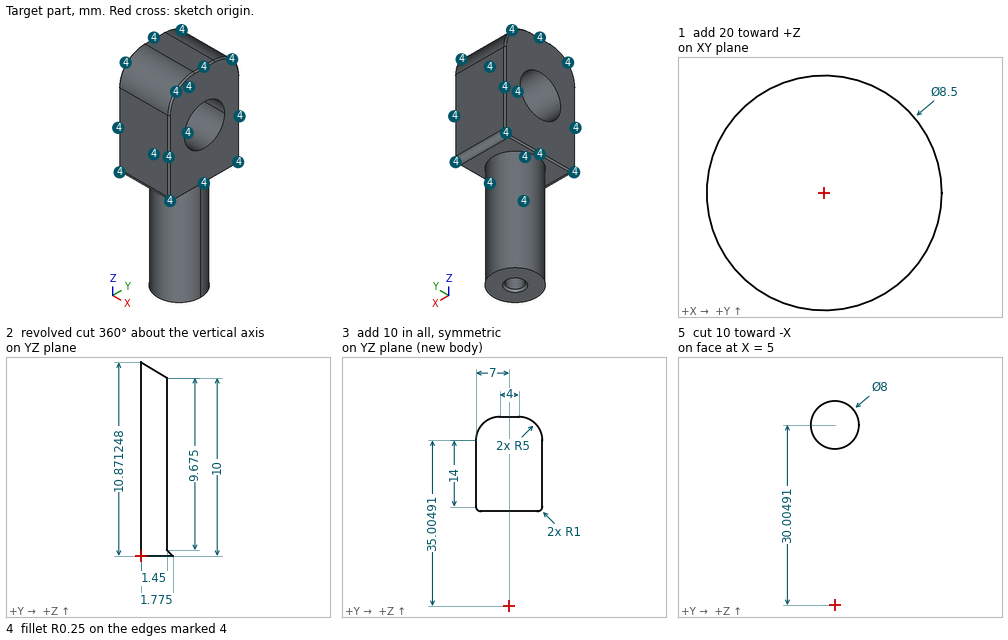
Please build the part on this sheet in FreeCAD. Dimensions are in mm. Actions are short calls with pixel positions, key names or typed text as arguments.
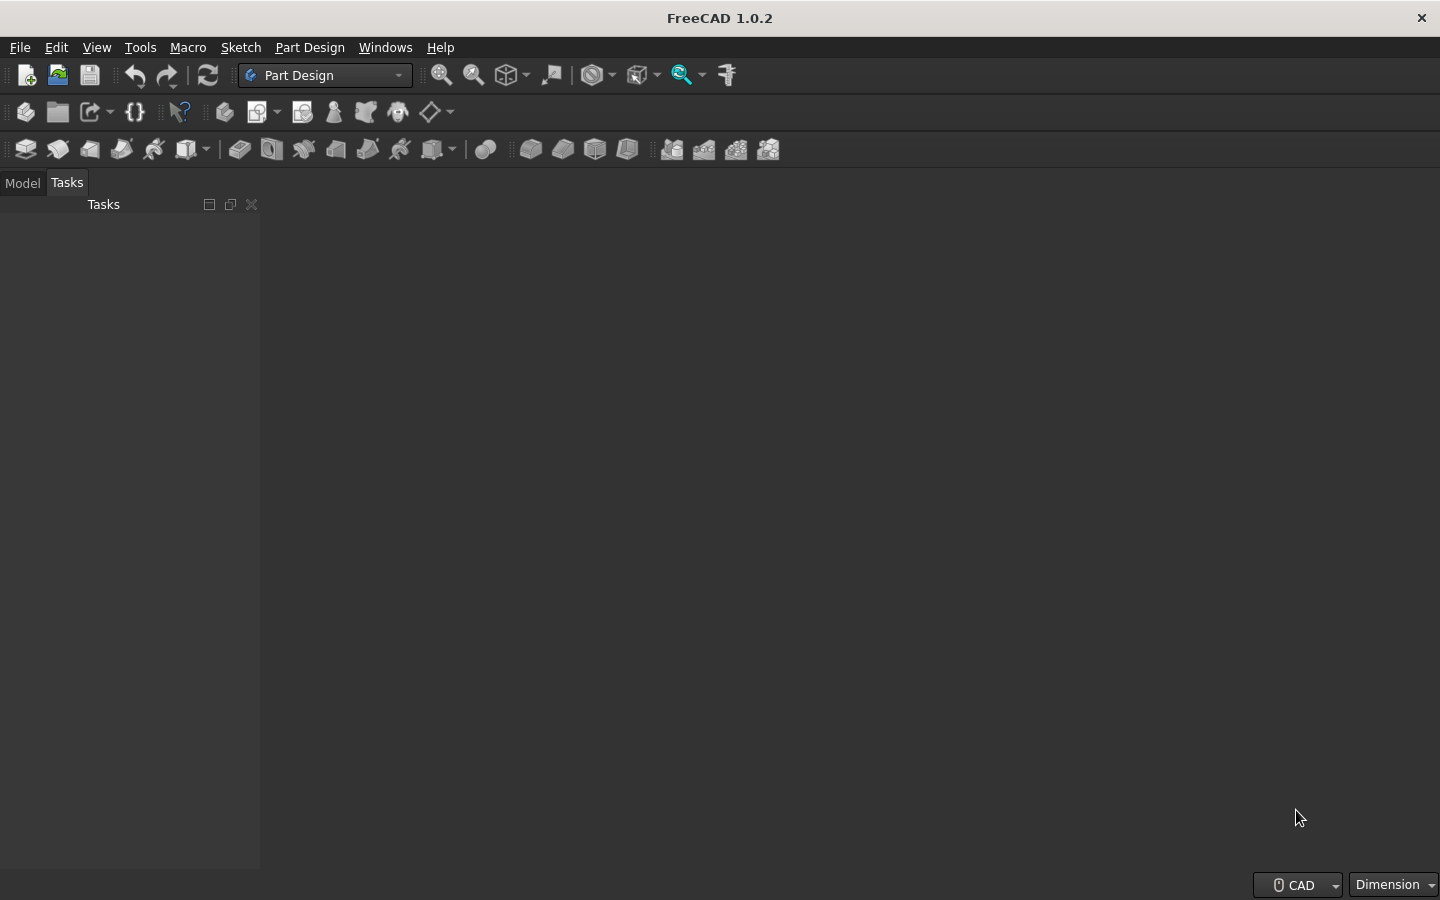
click(26, 76)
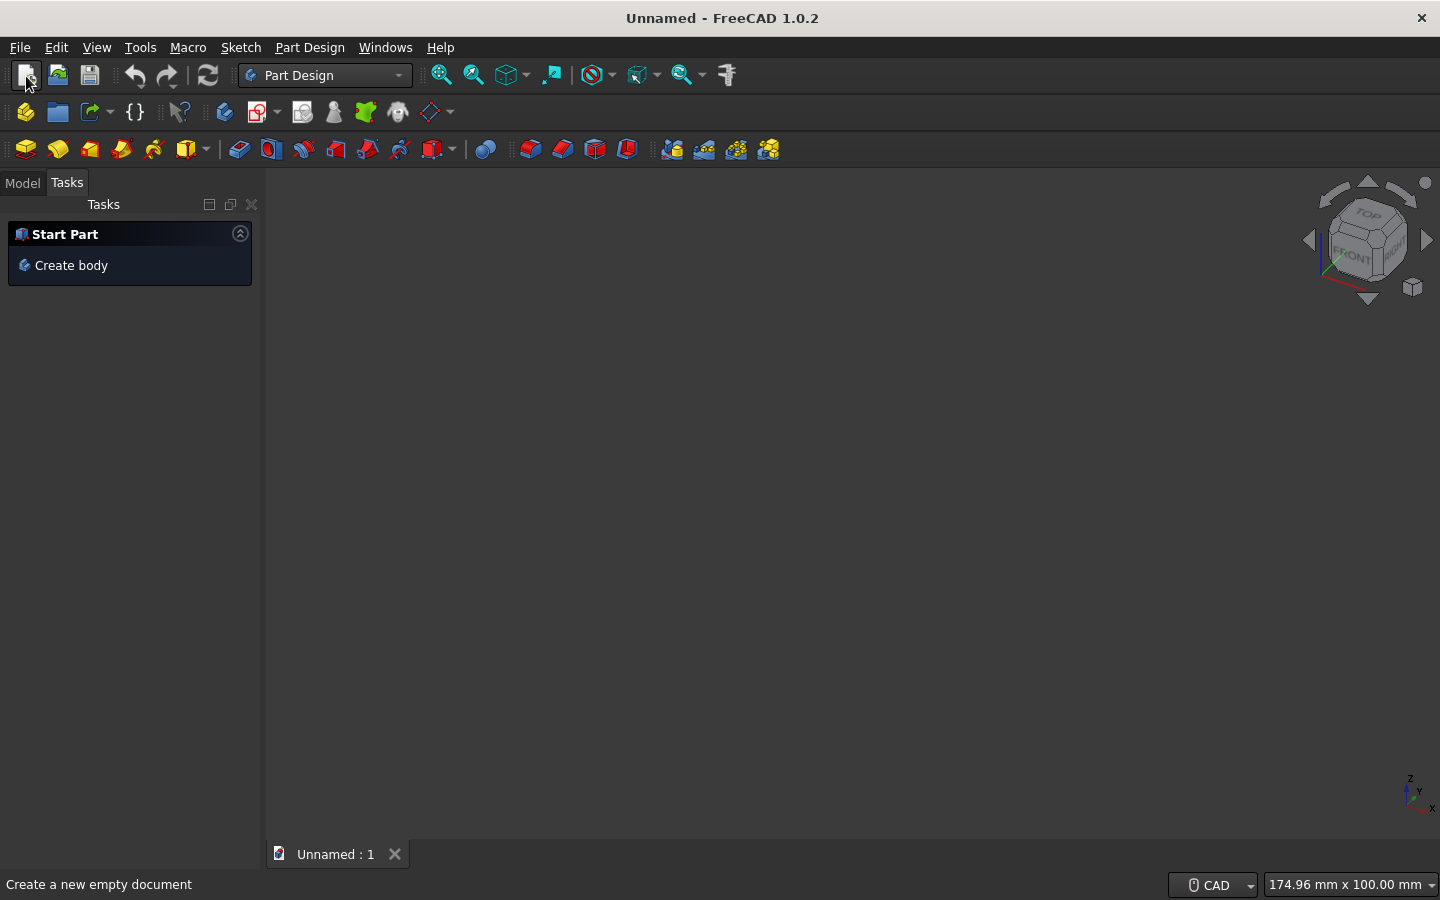
click(258, 112)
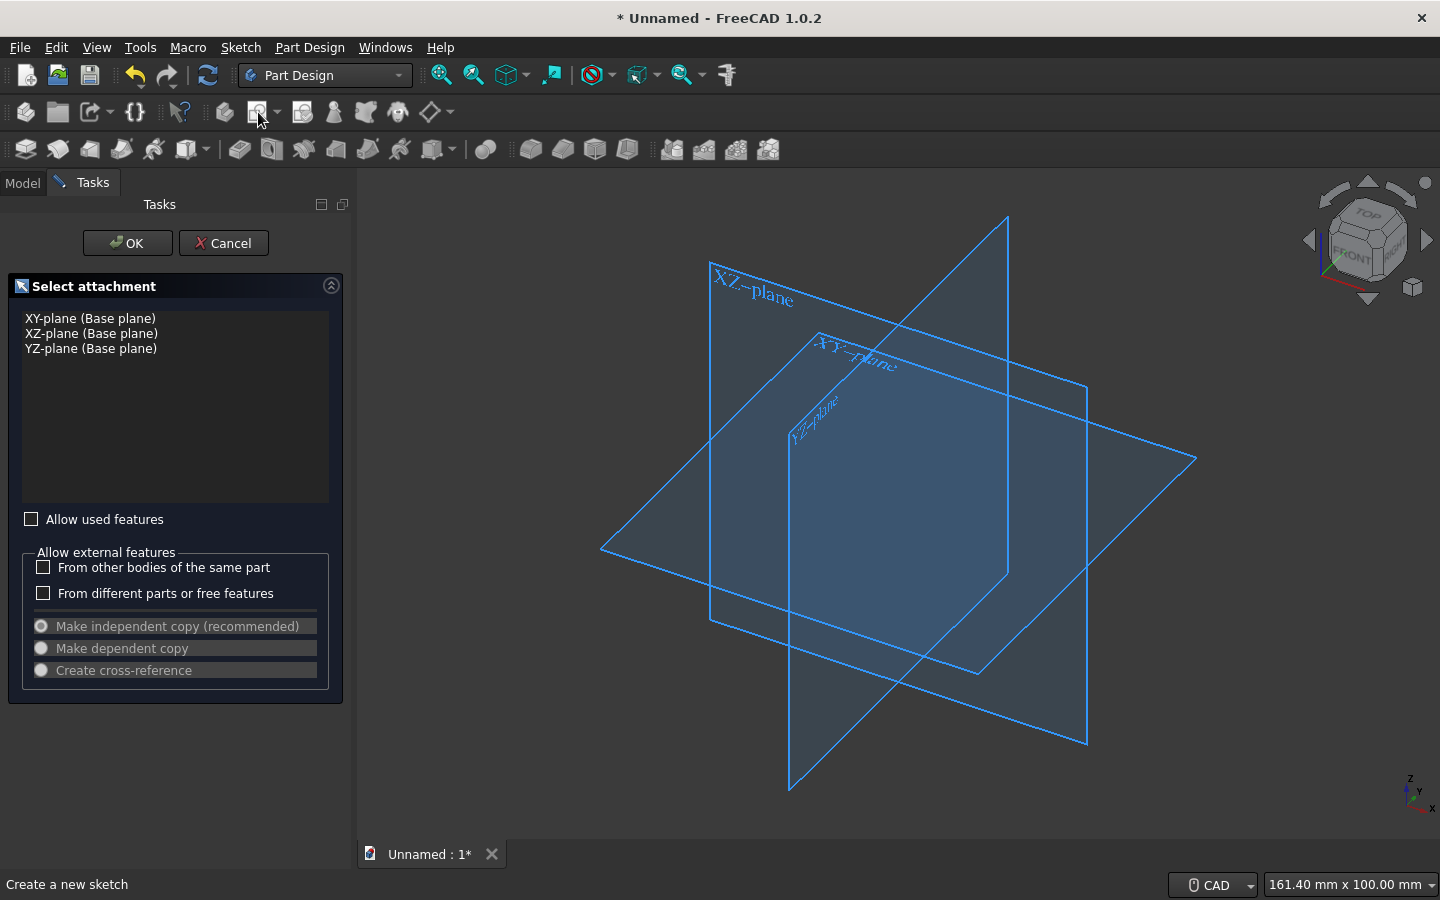
click(82, 318)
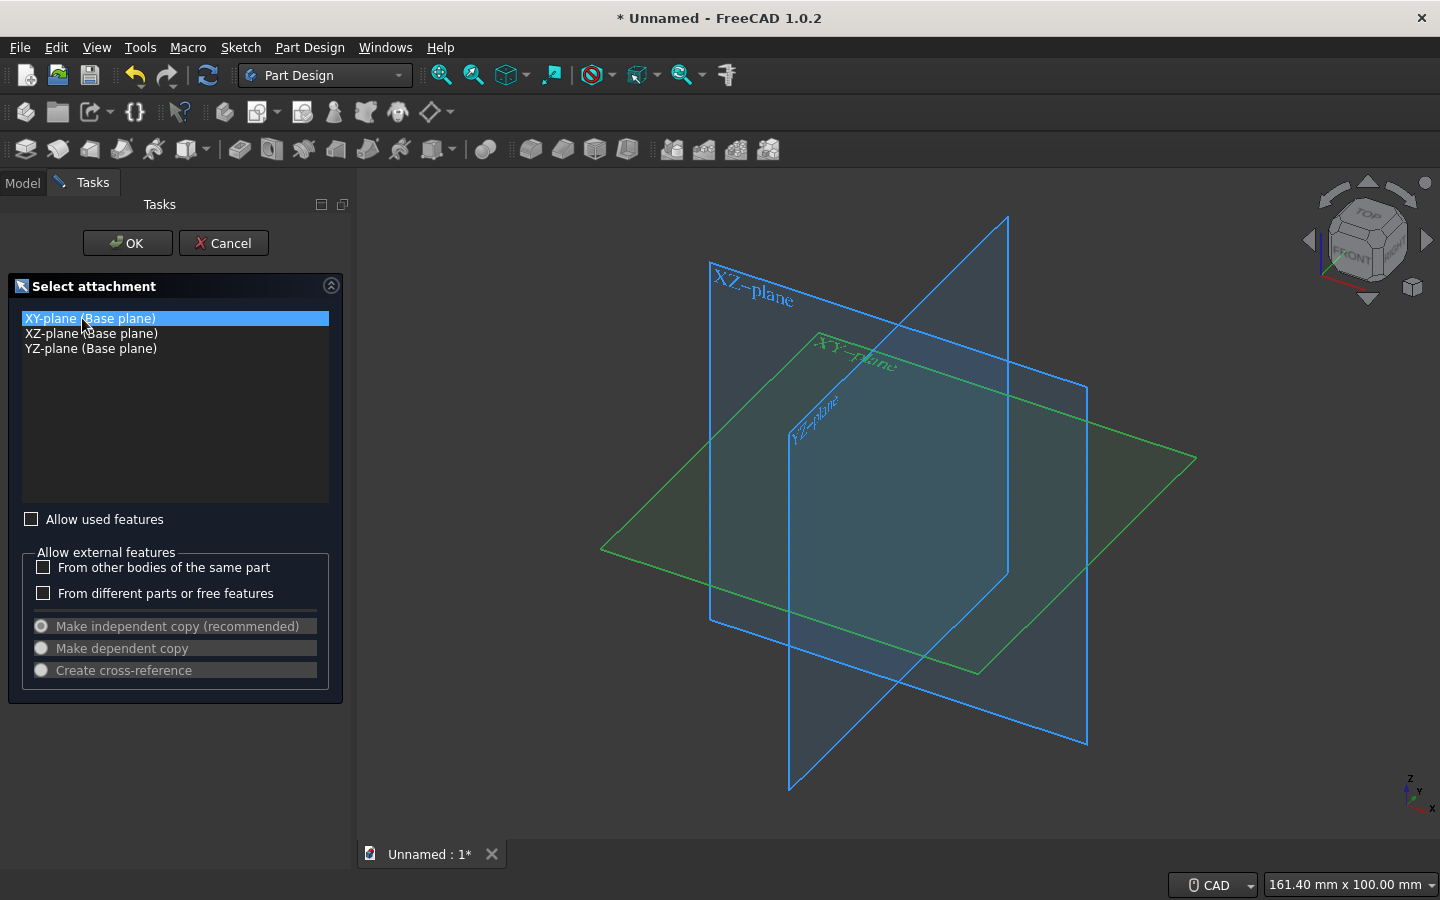
click(128, 243)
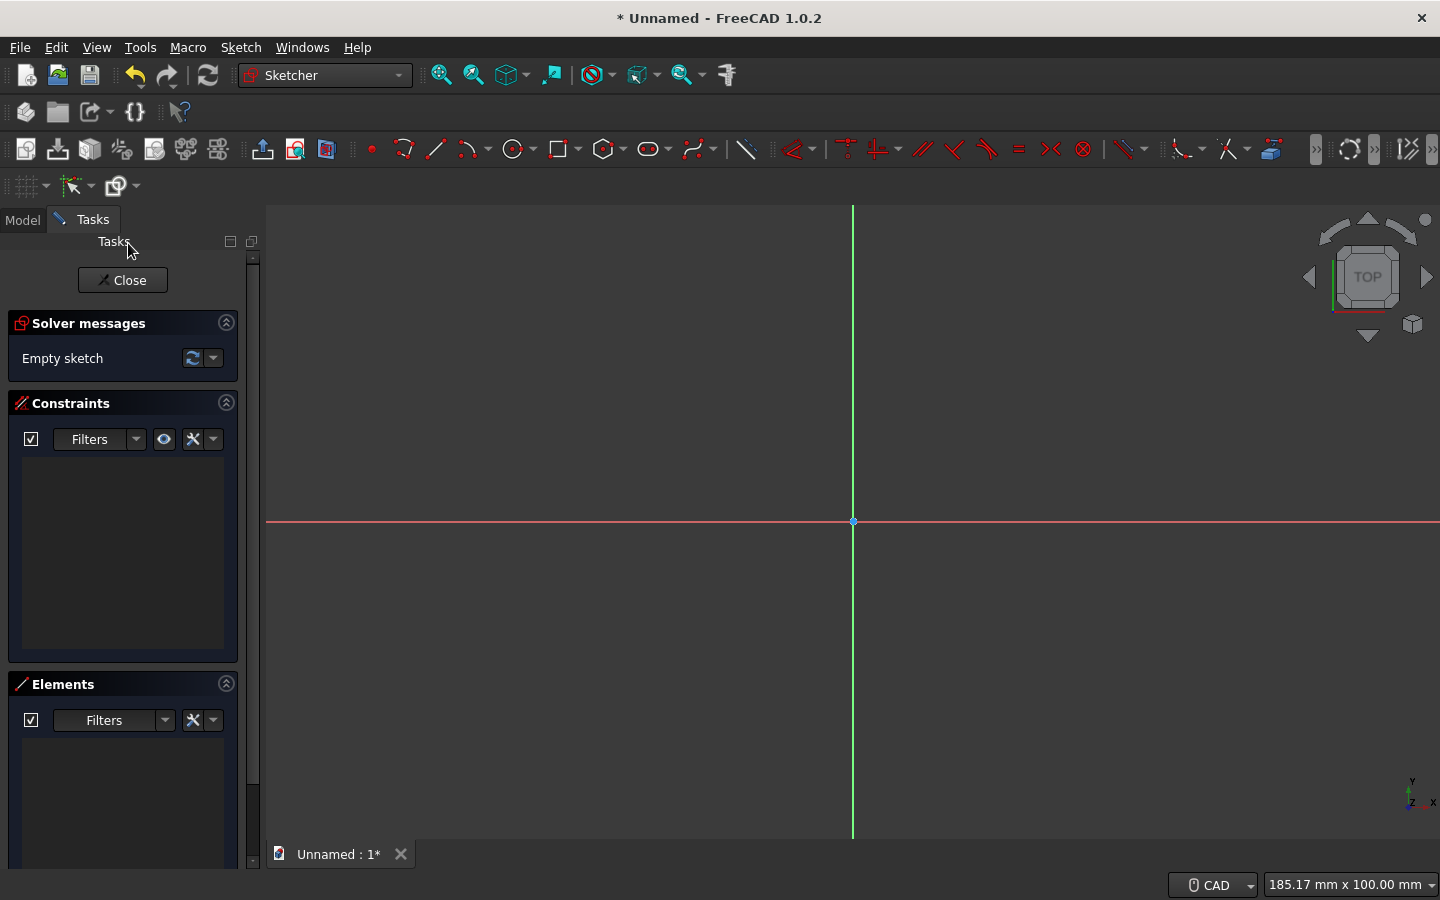
scroll(864, 522, up, 10)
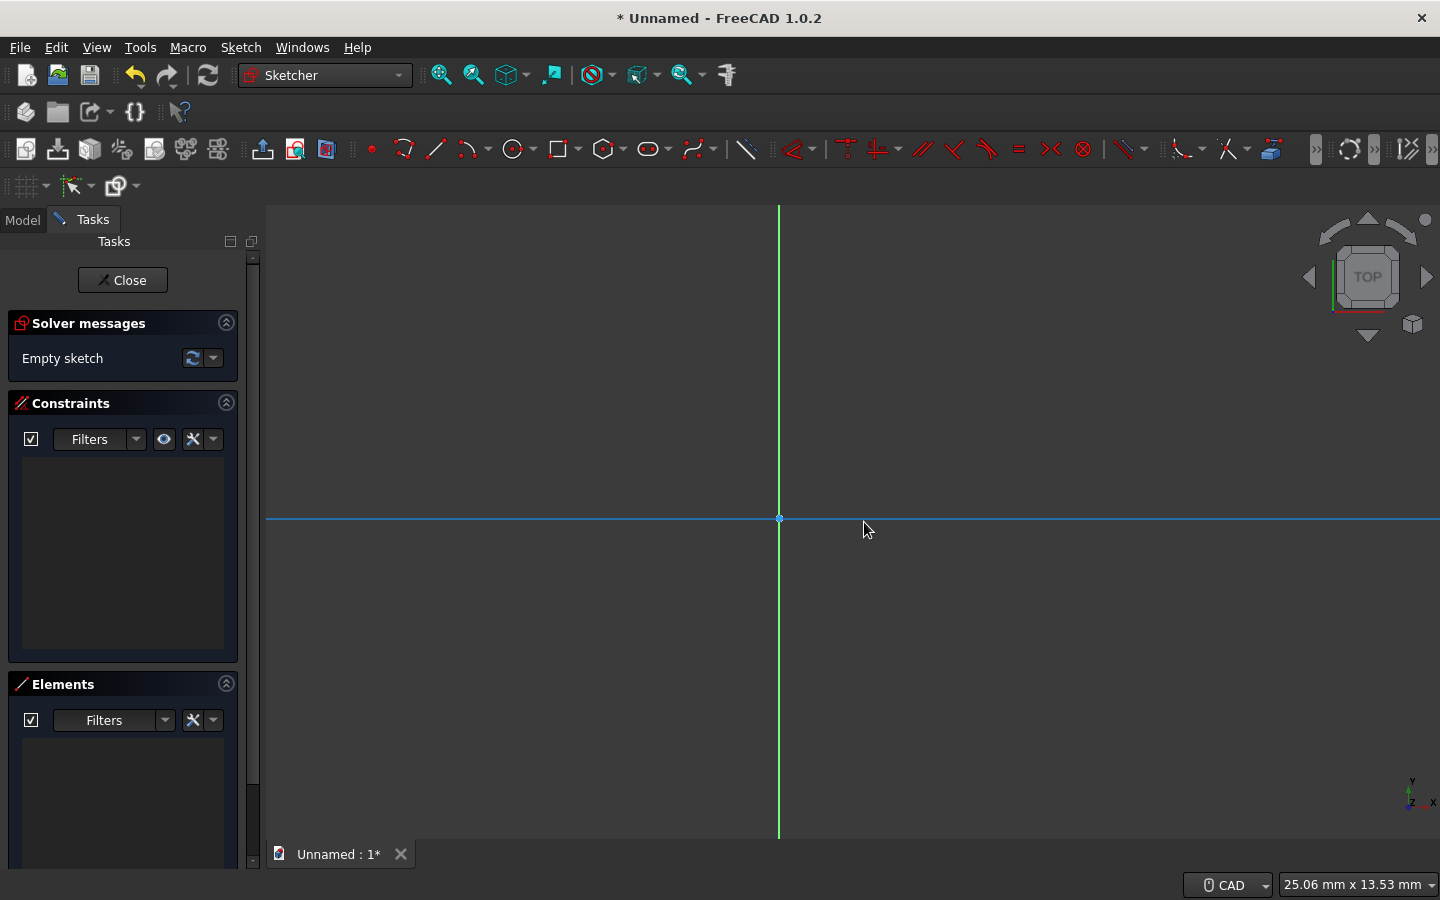
click(514, 150)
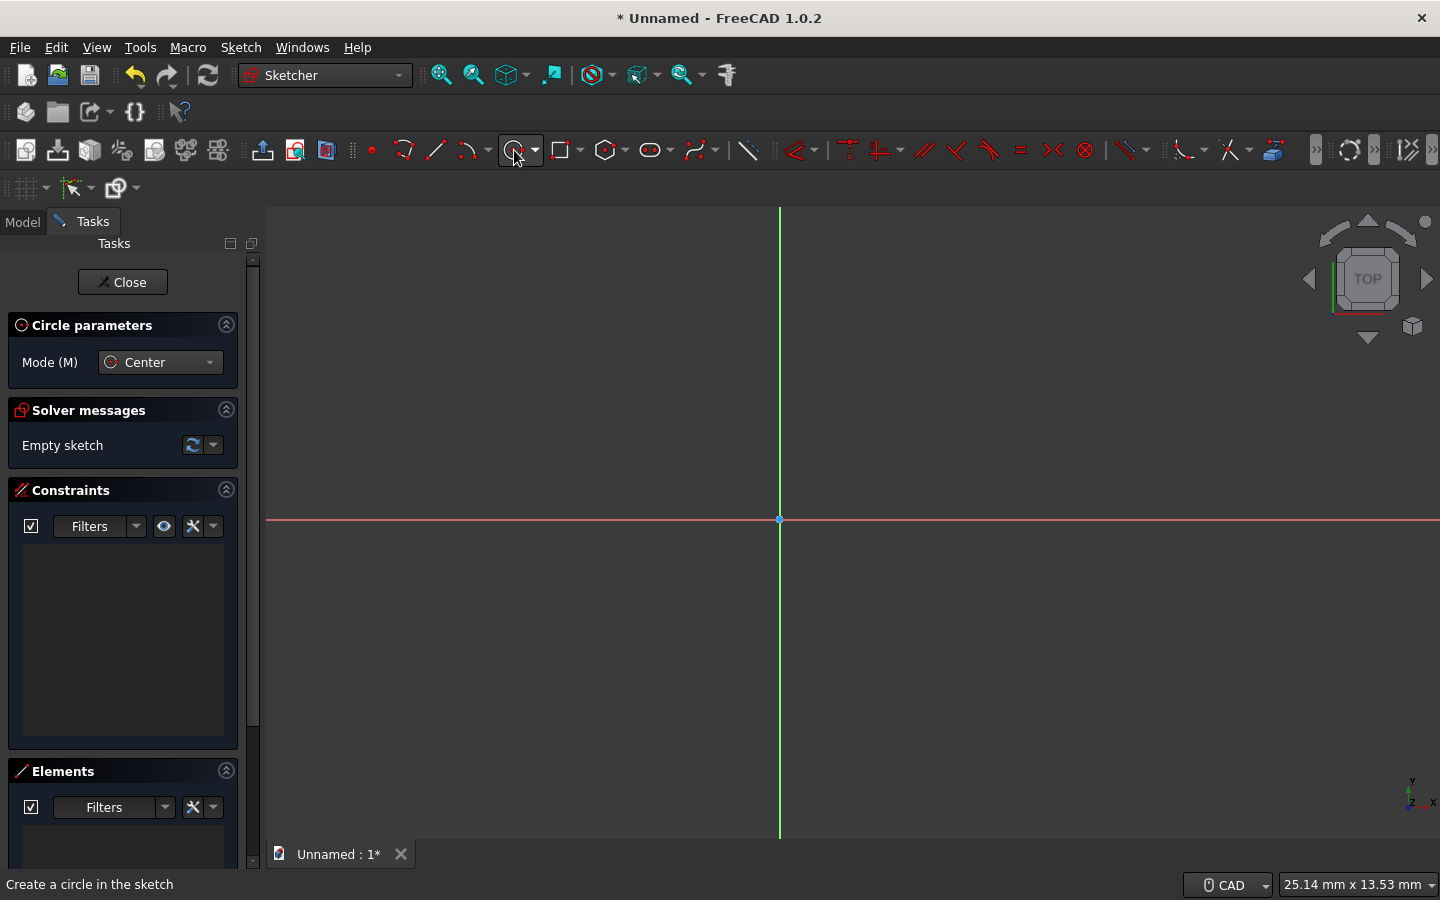
click(780, 520)
click(920, 379)
key(Escape)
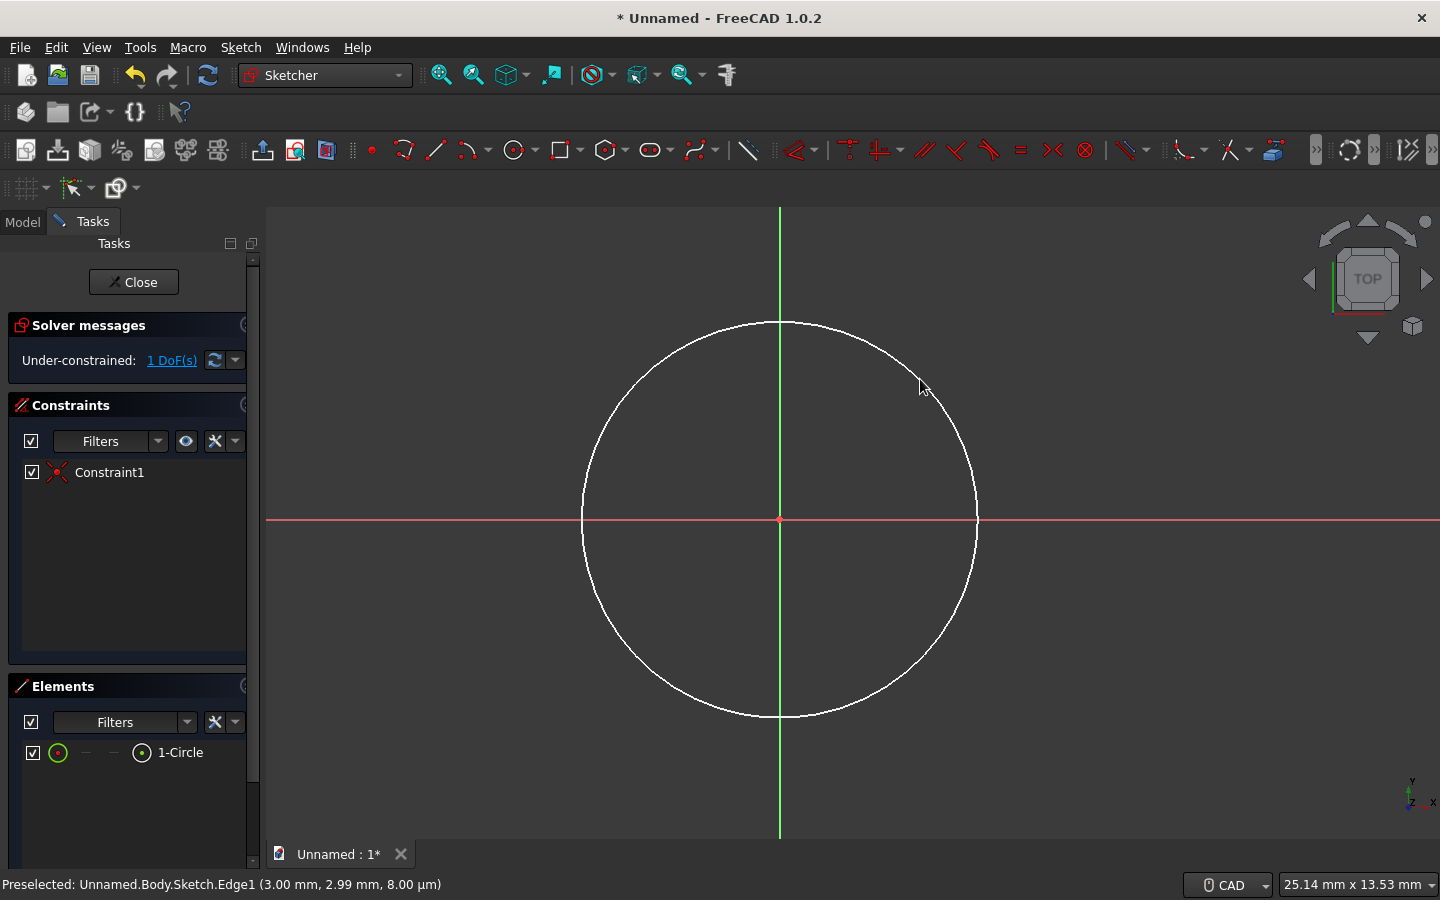
click(794, 150)